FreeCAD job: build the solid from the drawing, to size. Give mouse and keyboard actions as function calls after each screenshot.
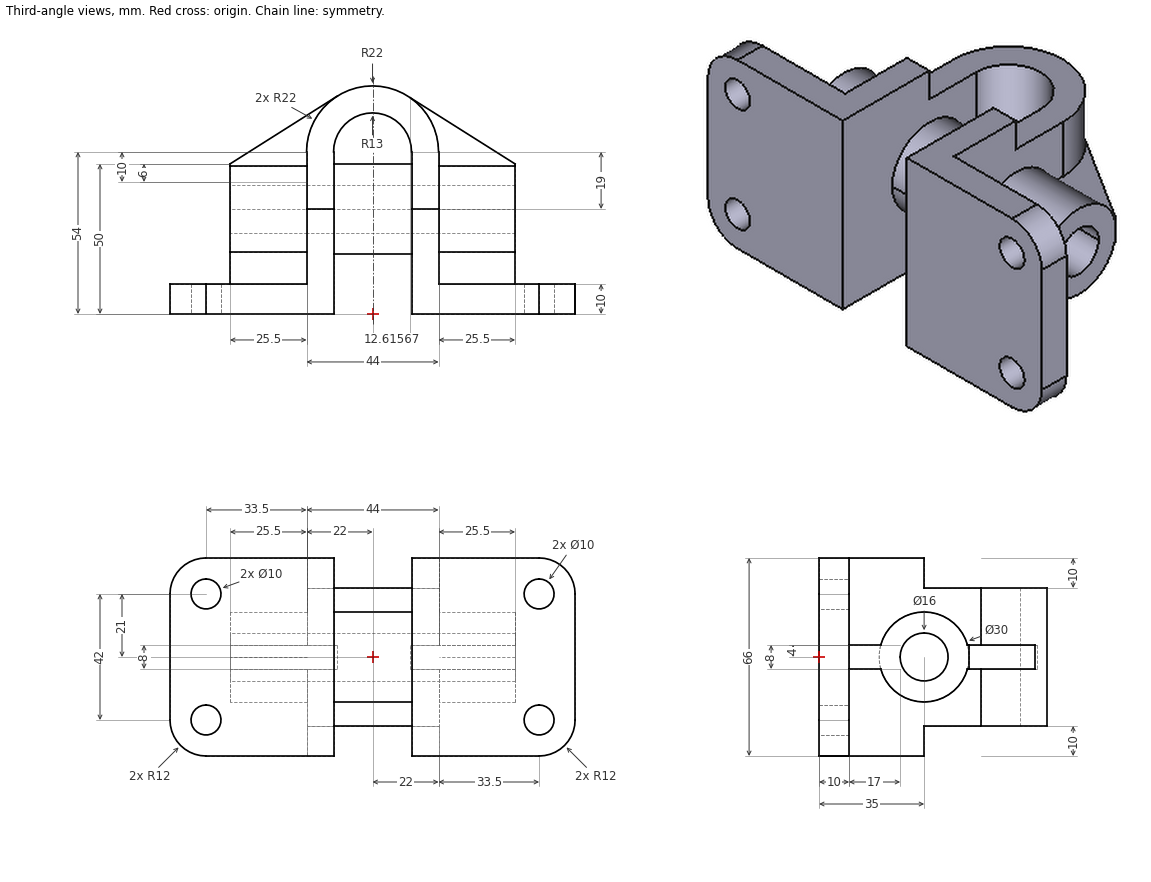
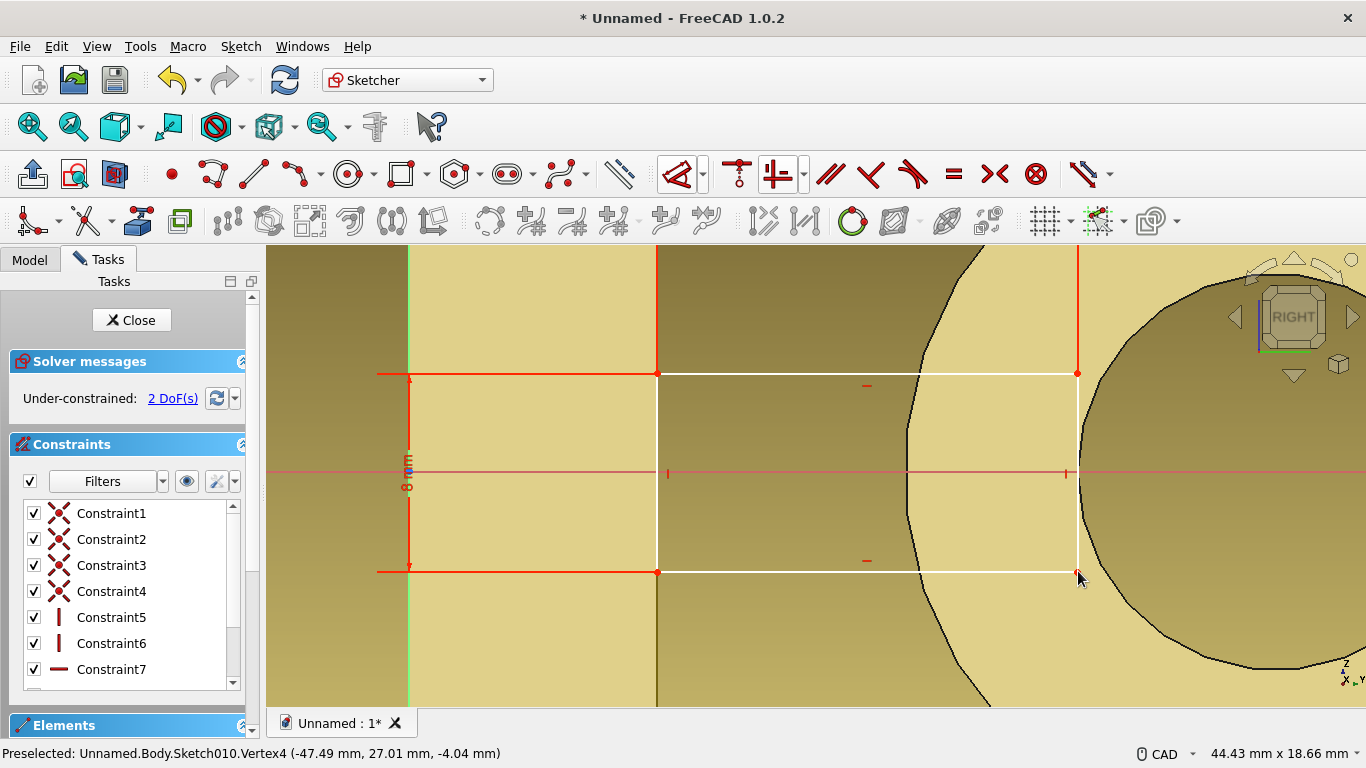
click(657, 374)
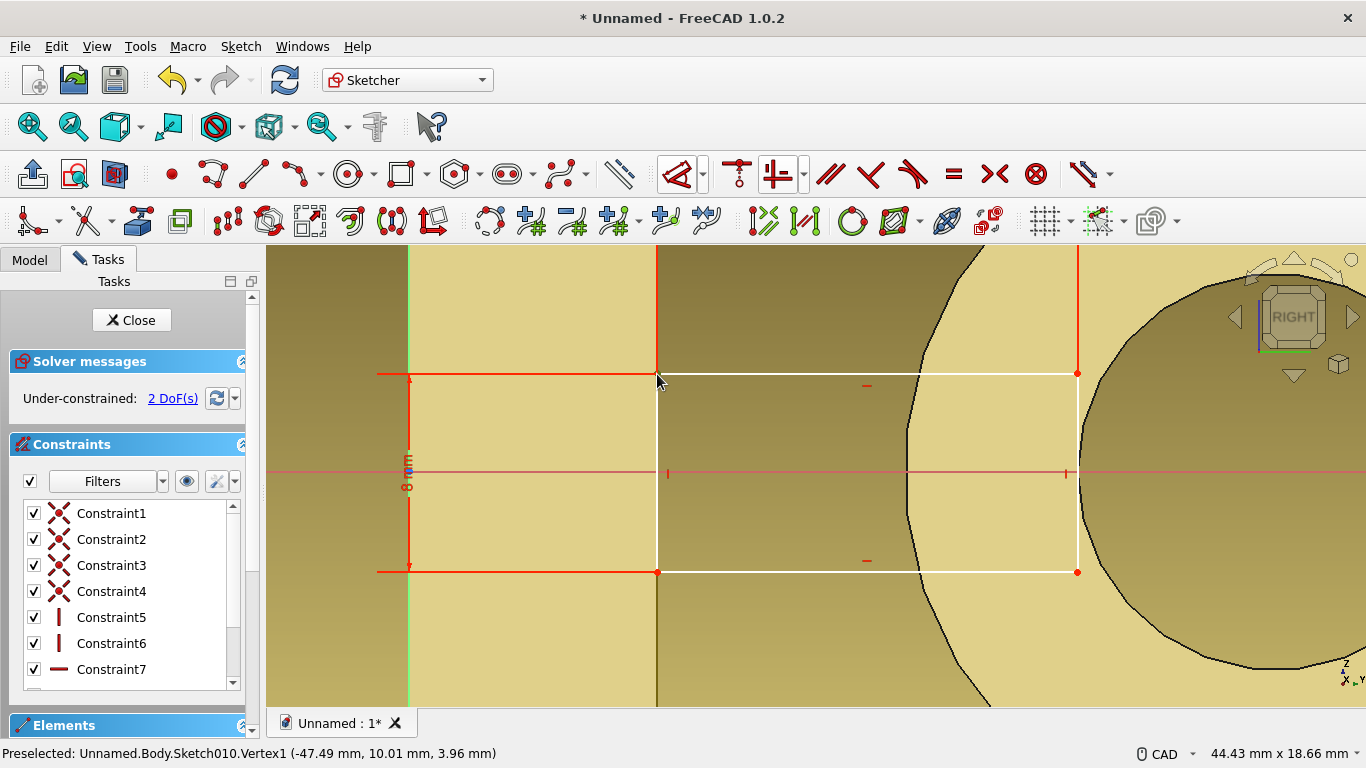
click(702, 174)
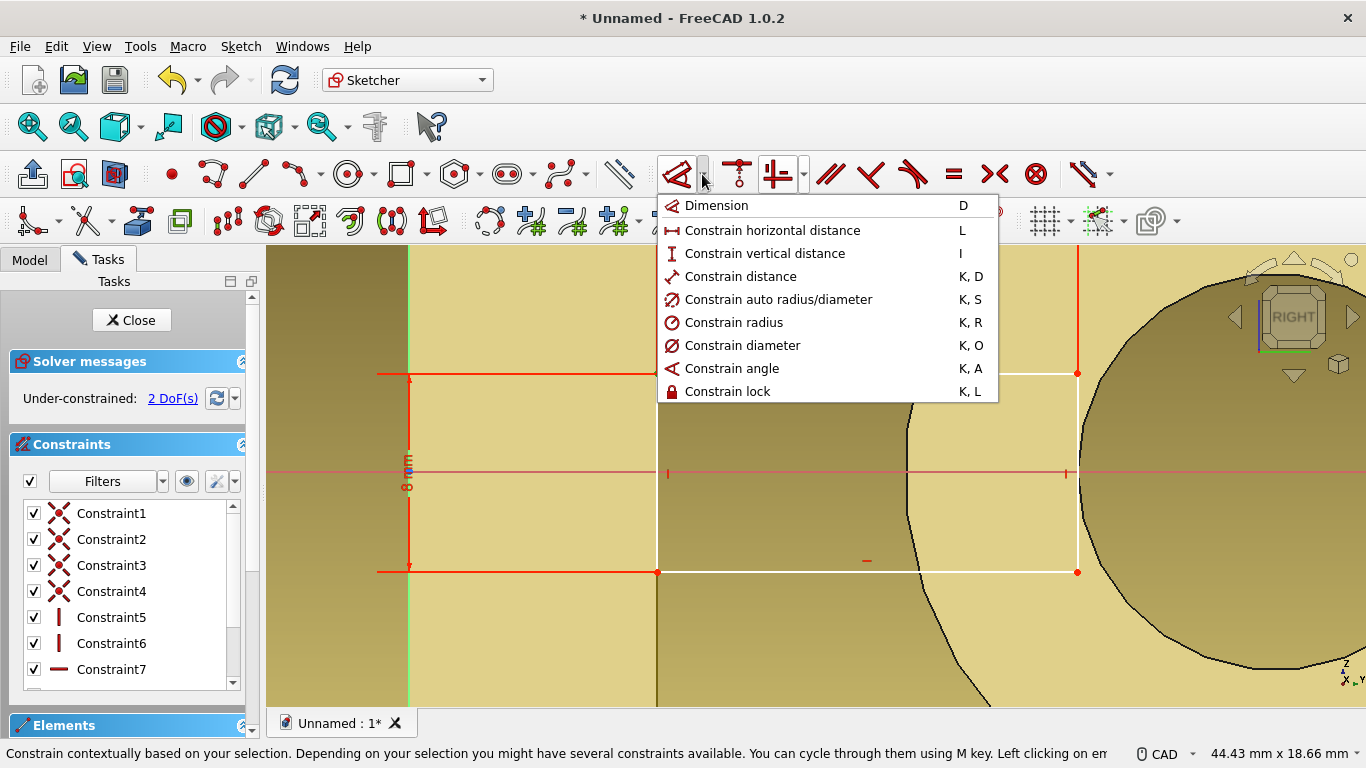
click(828, 254)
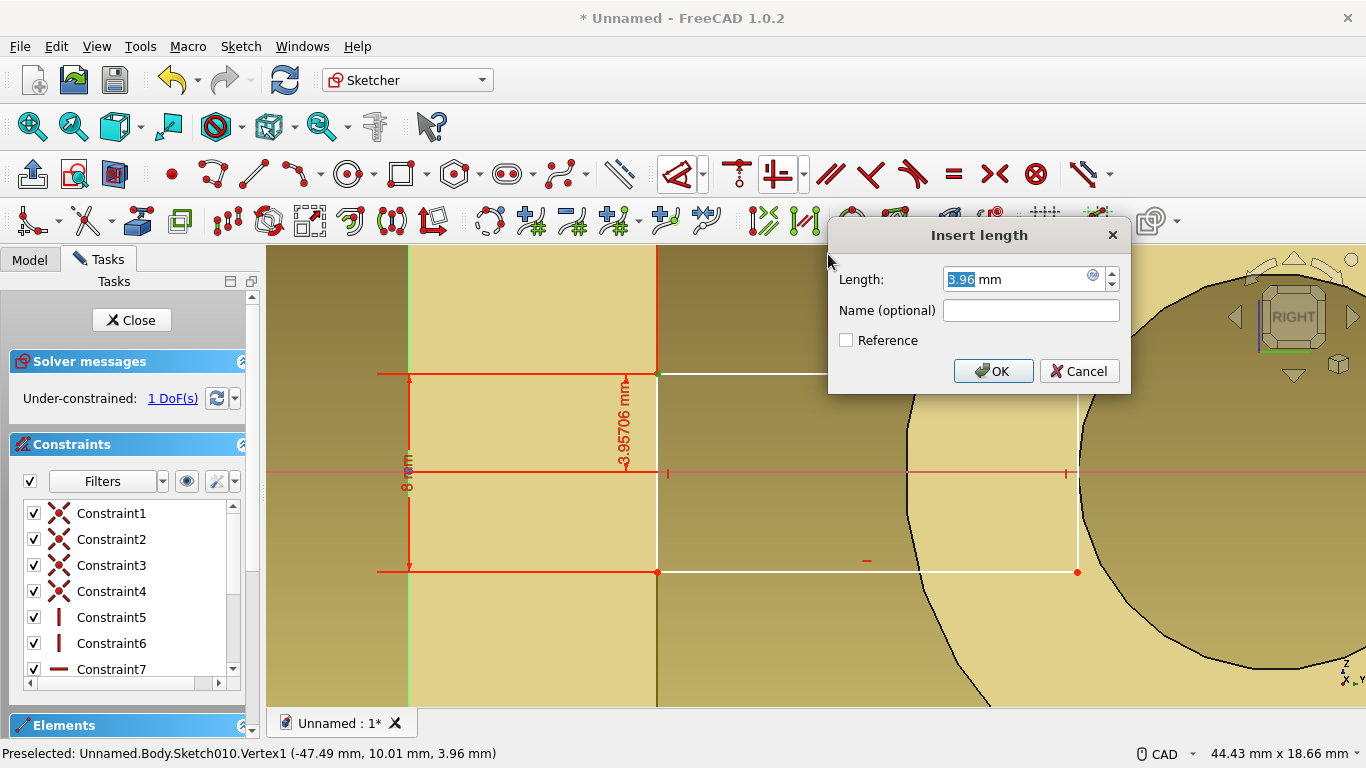
text(4)
key(Return)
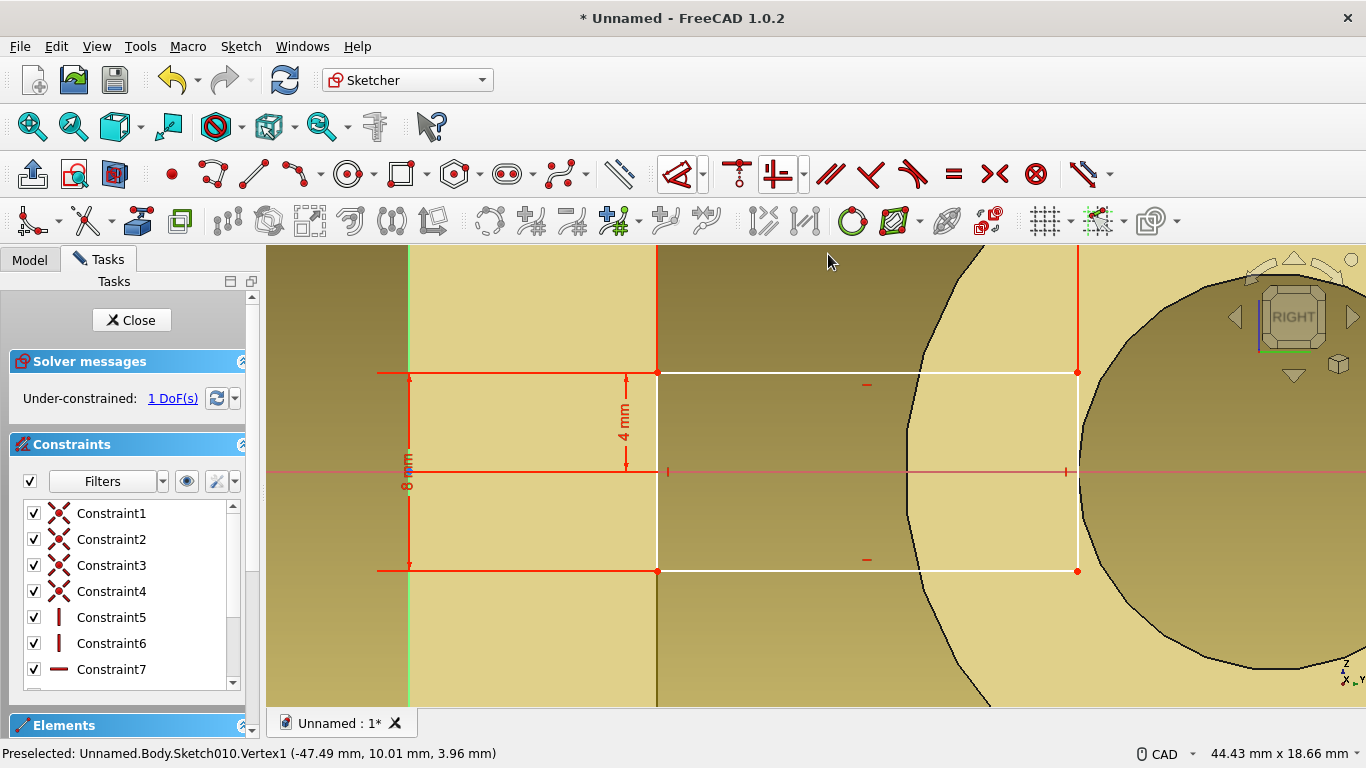
click(657, 373)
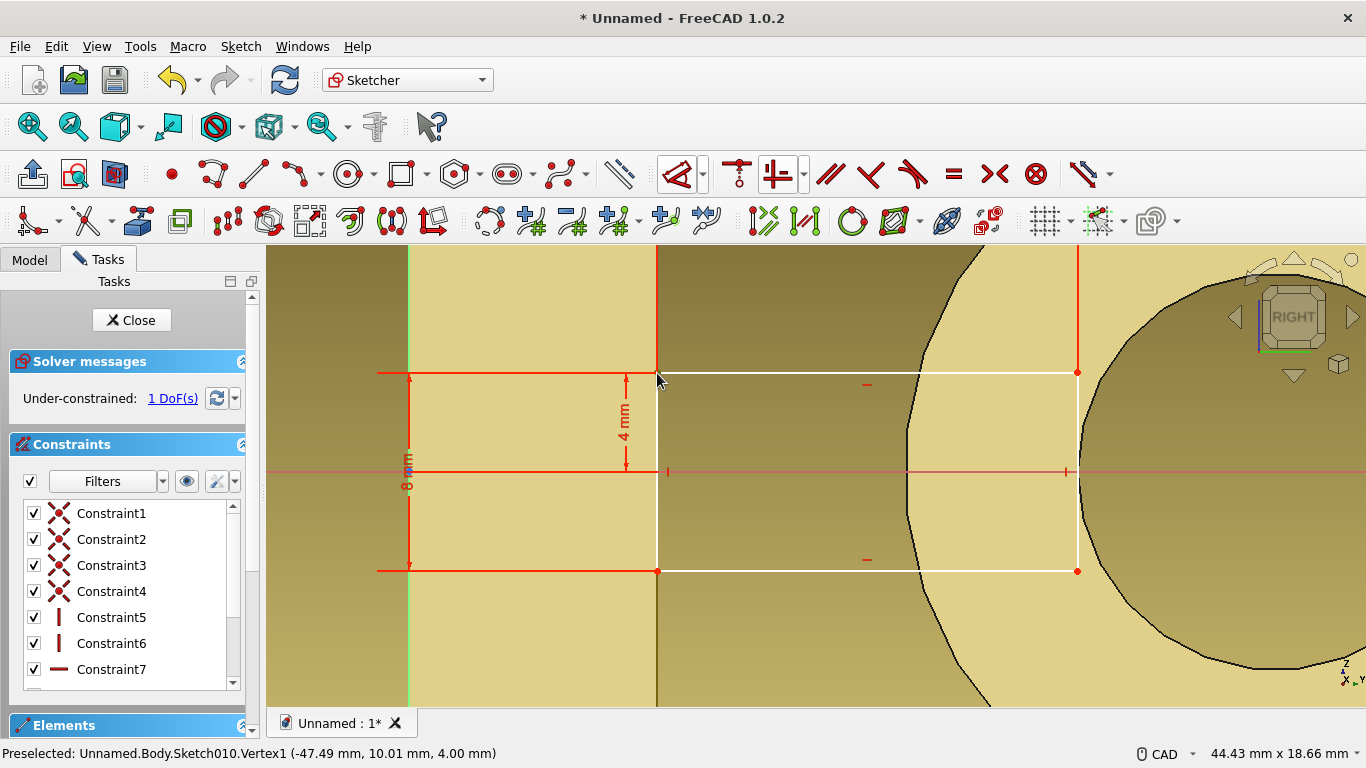
key(l)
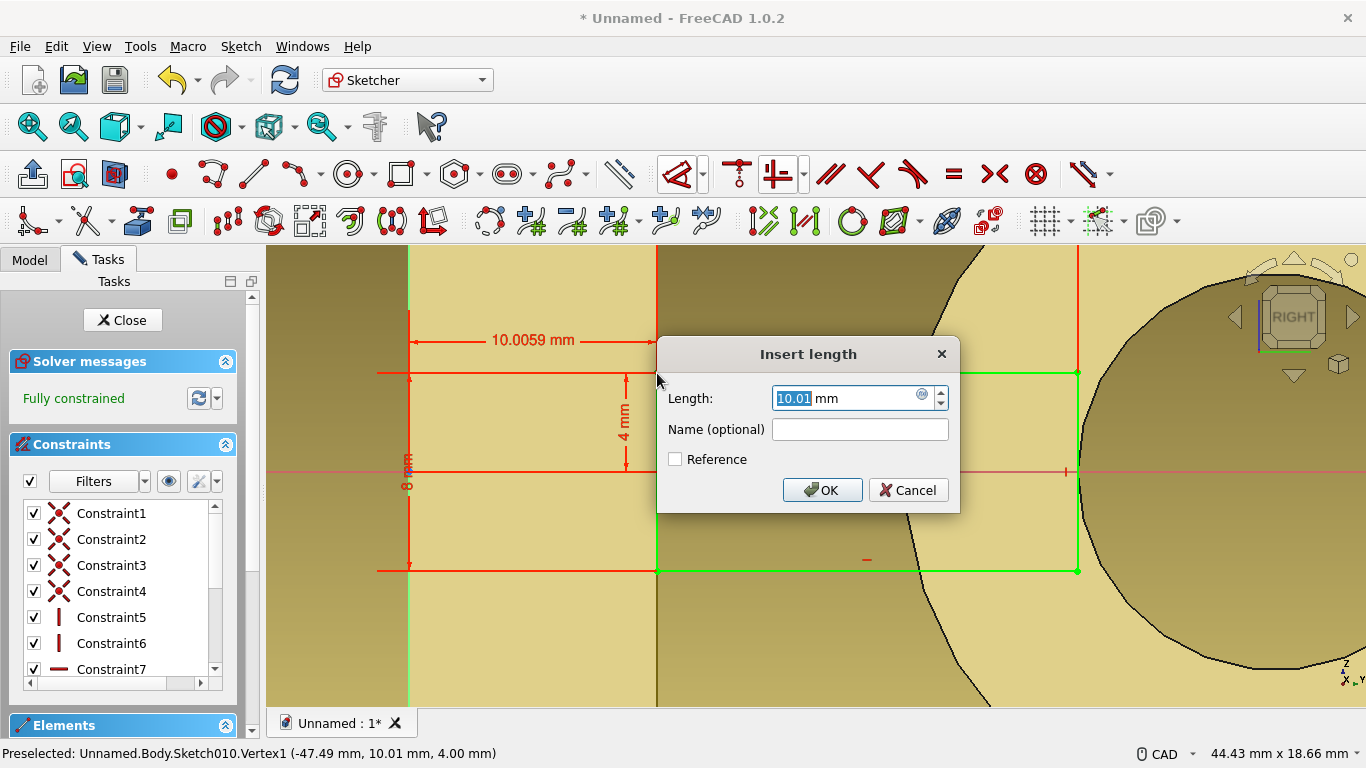
text(10)
key(Return)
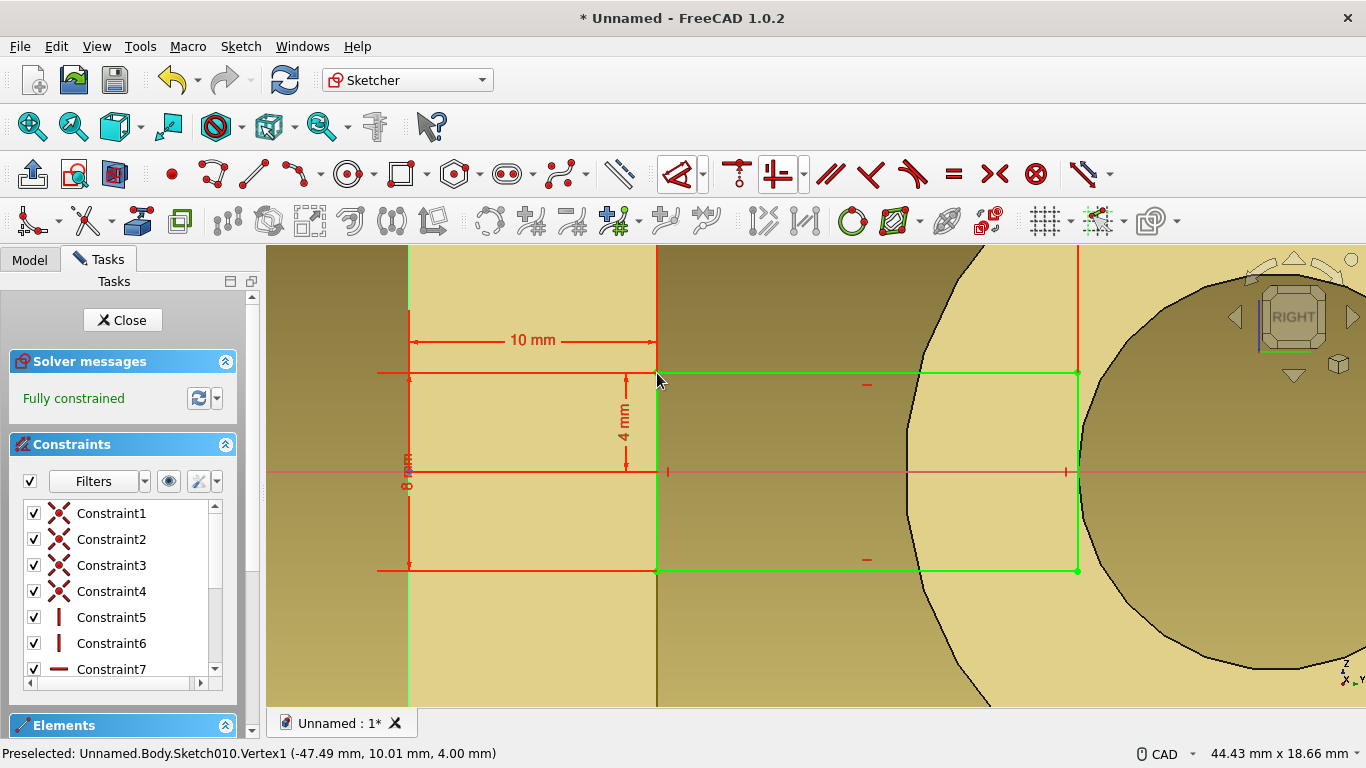
click(123, 320)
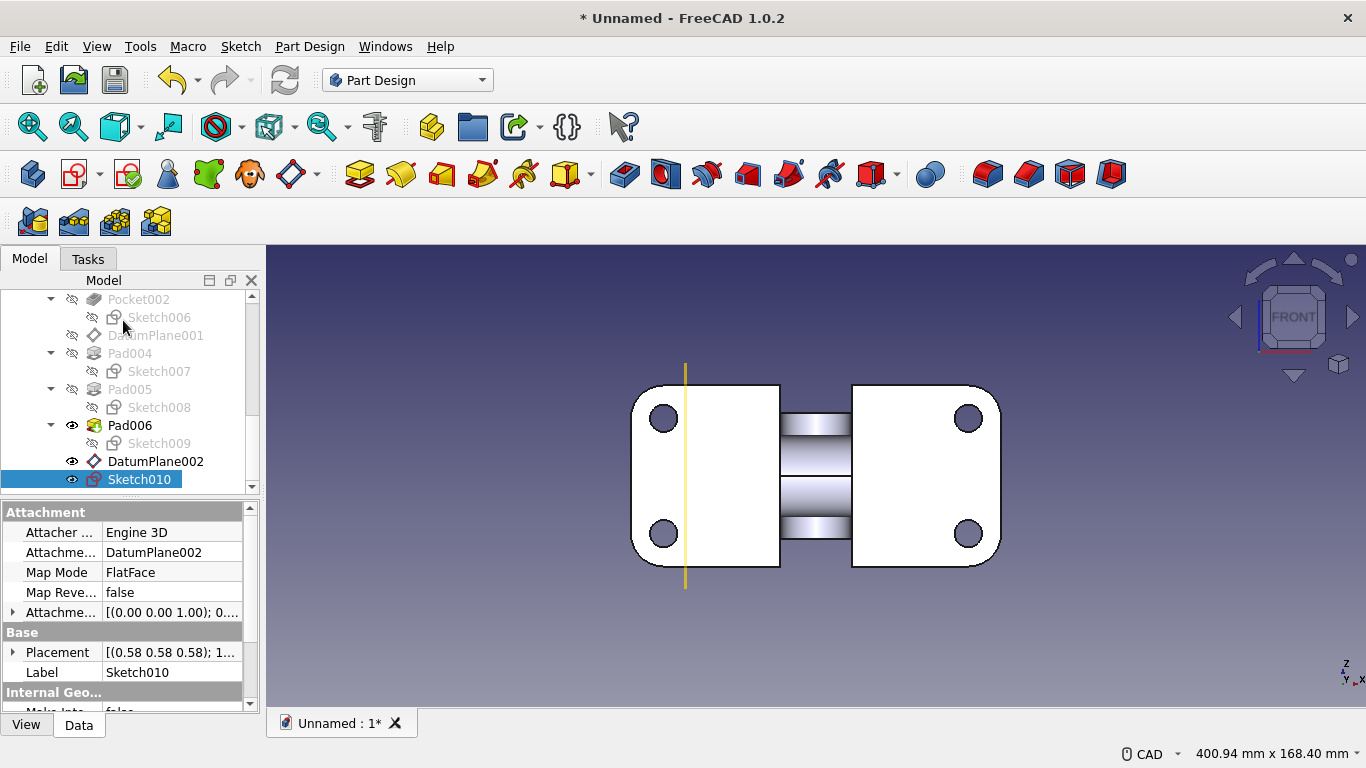
click(360, 174)